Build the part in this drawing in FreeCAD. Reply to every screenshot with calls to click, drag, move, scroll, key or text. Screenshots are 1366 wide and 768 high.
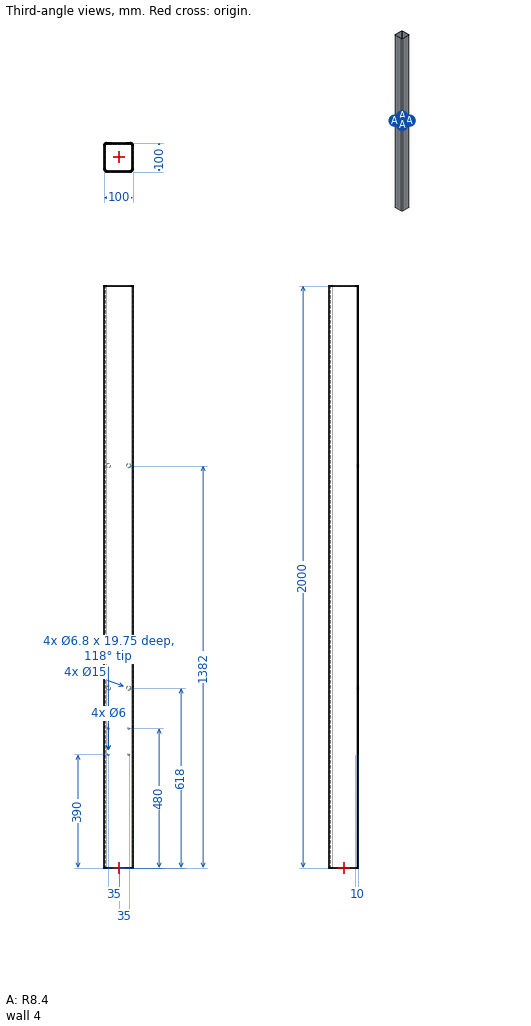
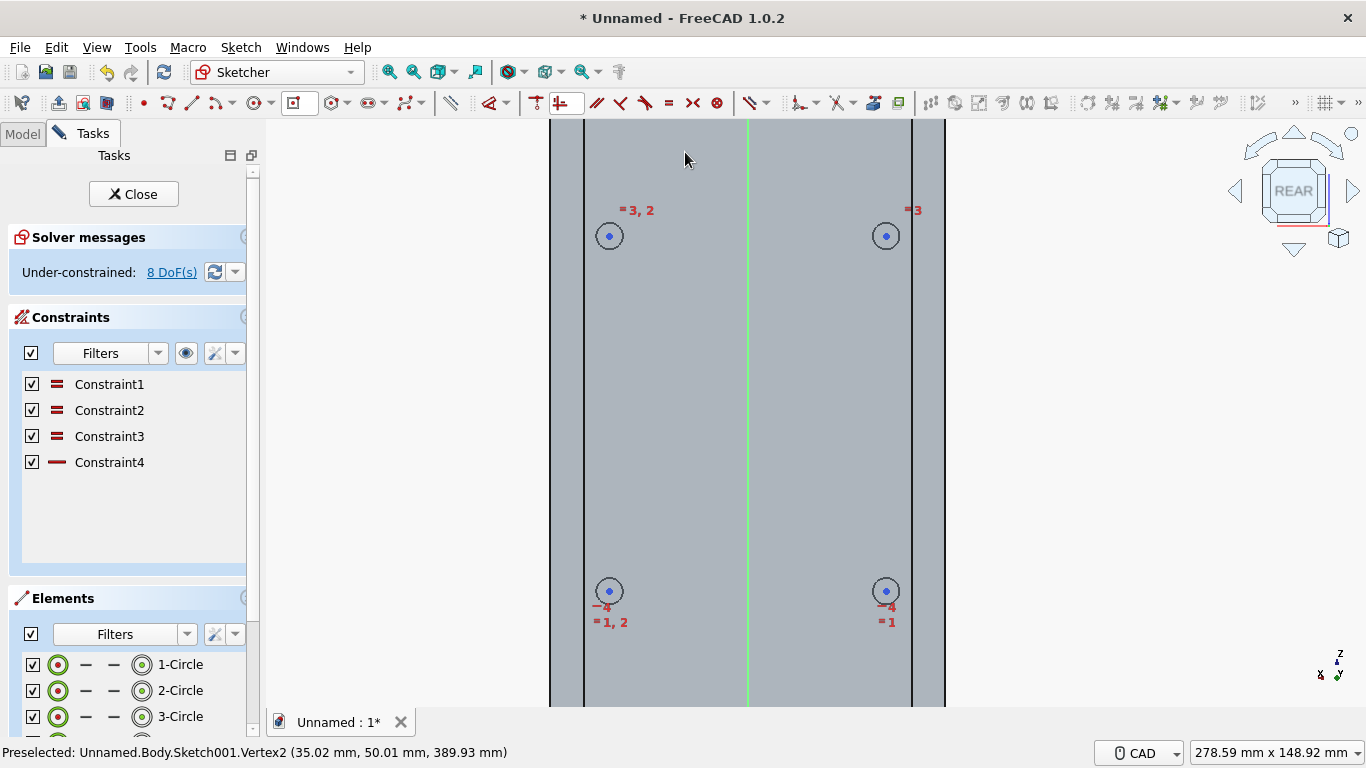
click(610, 591)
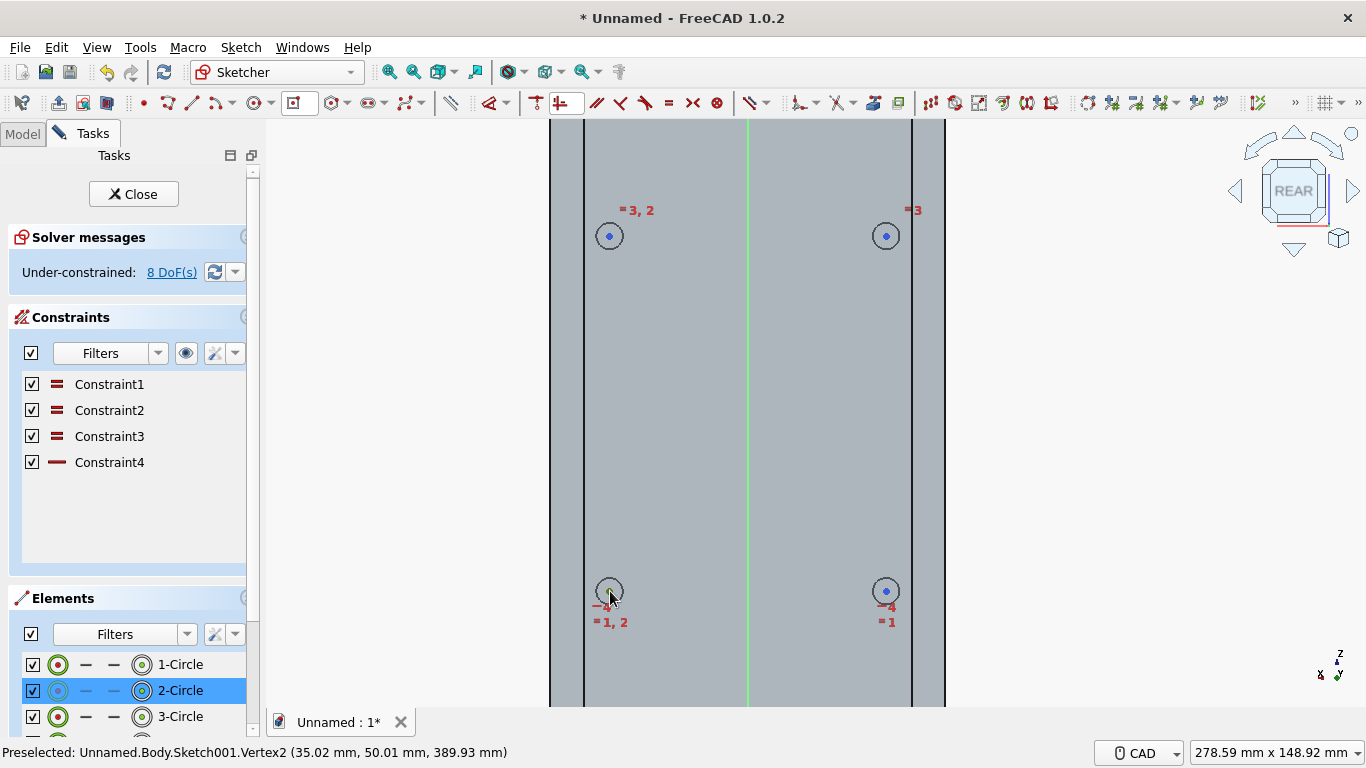
click(610, 236)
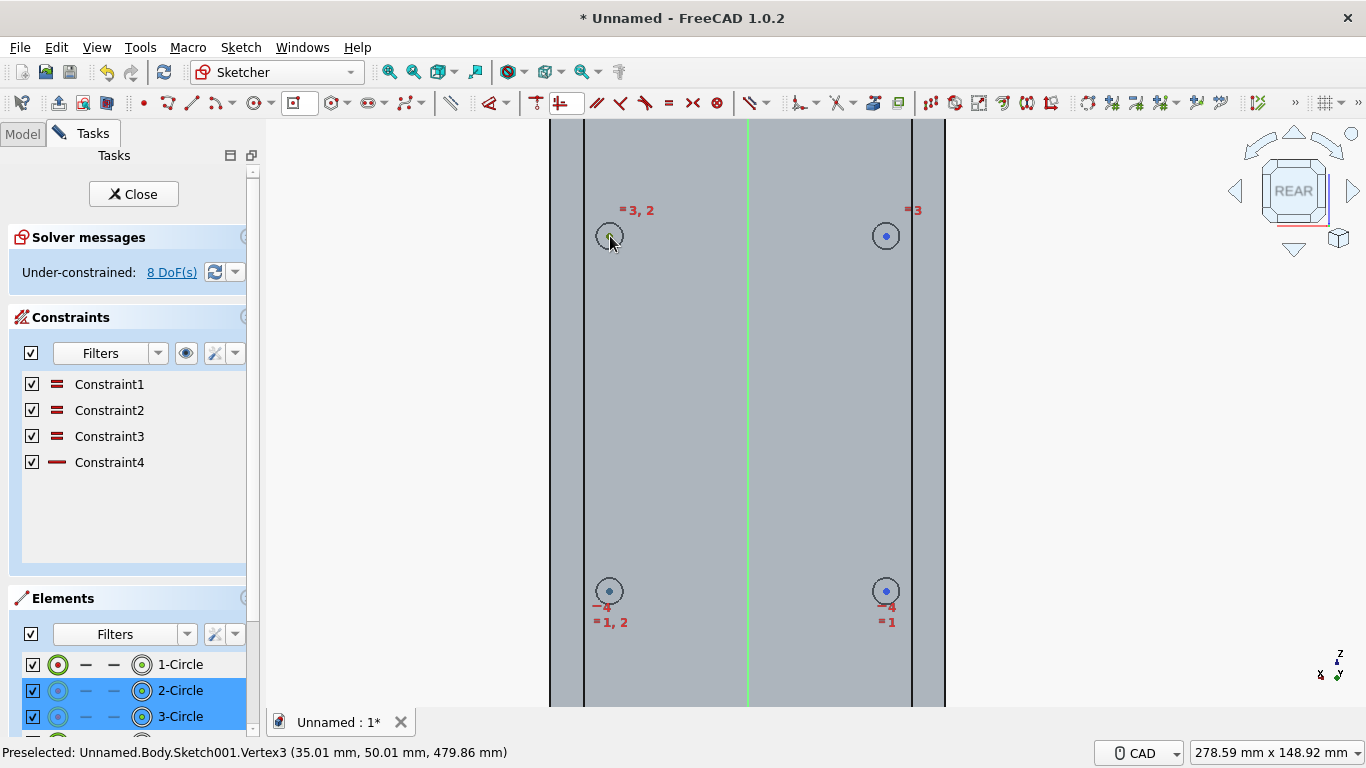
click(578, 104)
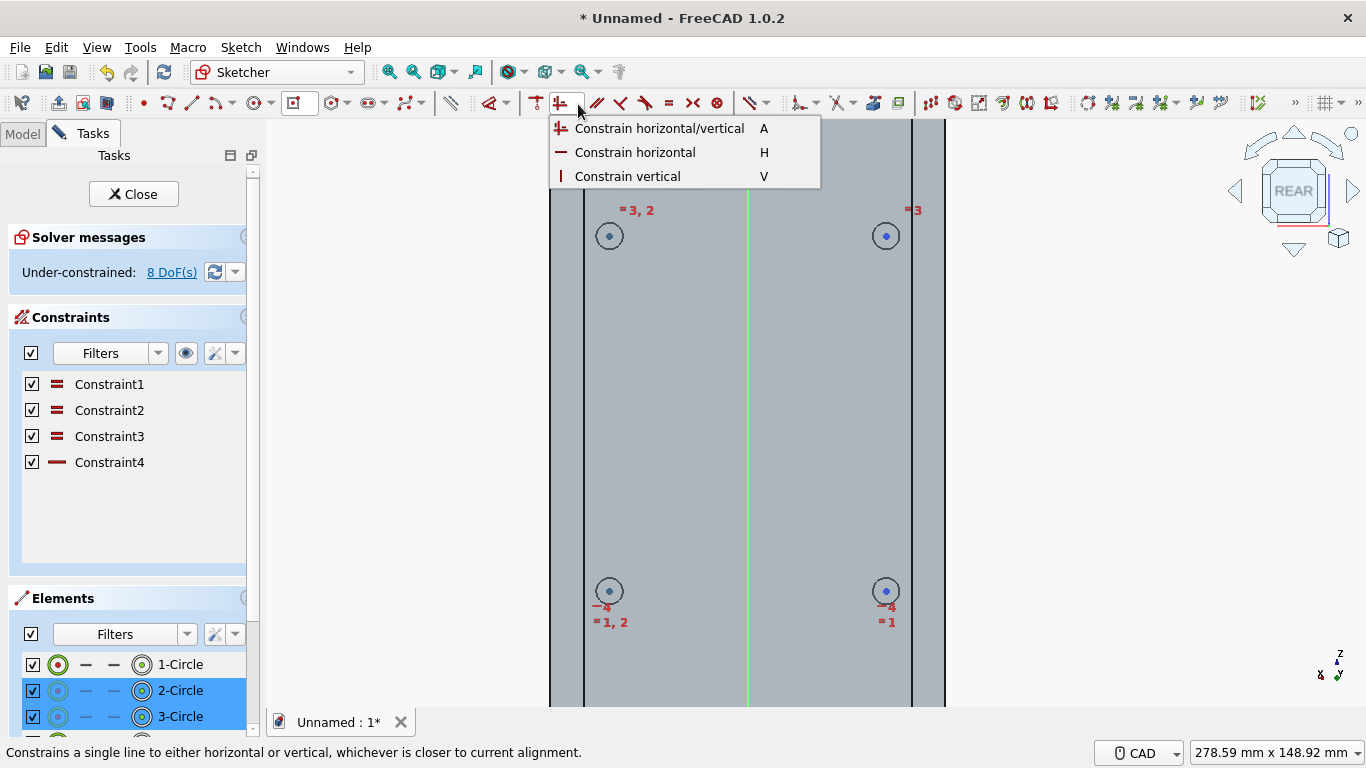
click(685, 176)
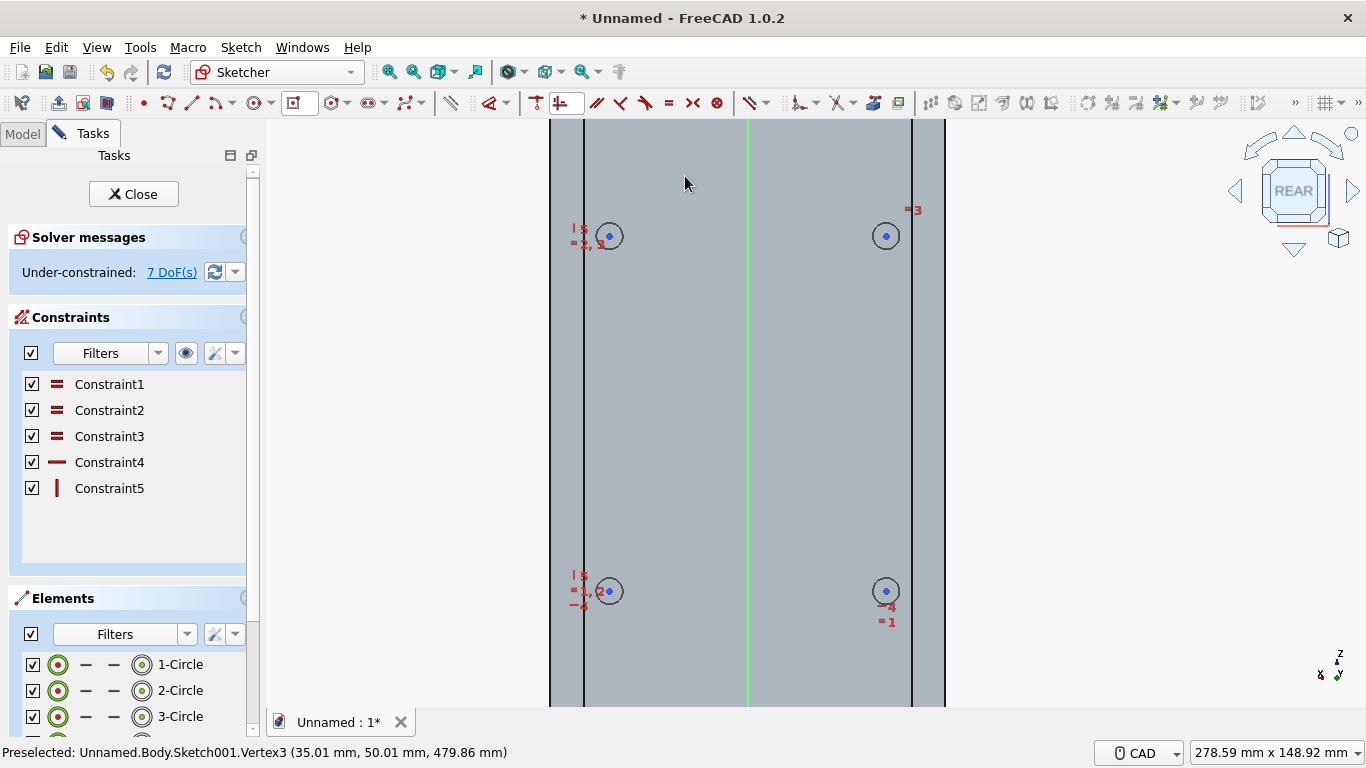
click(886, 591)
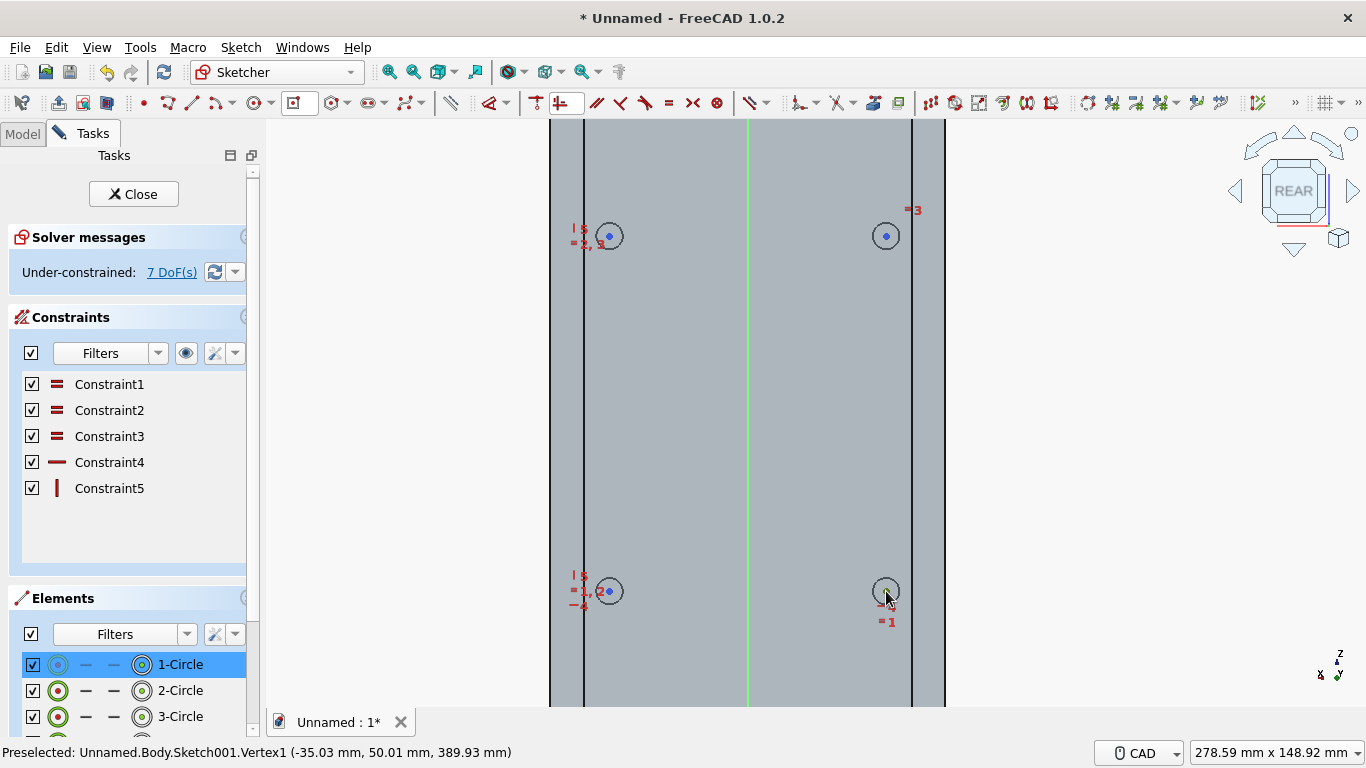
click(886, 236)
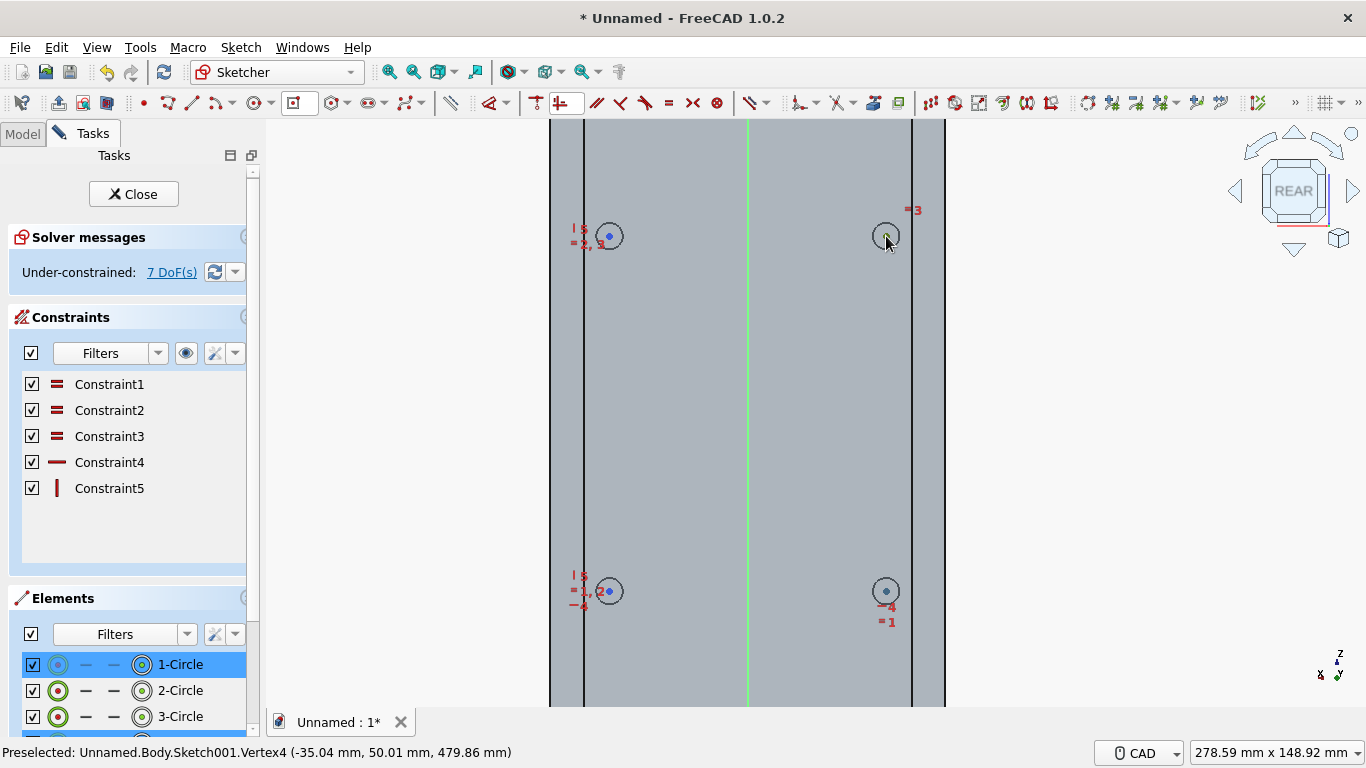
click(578, 104)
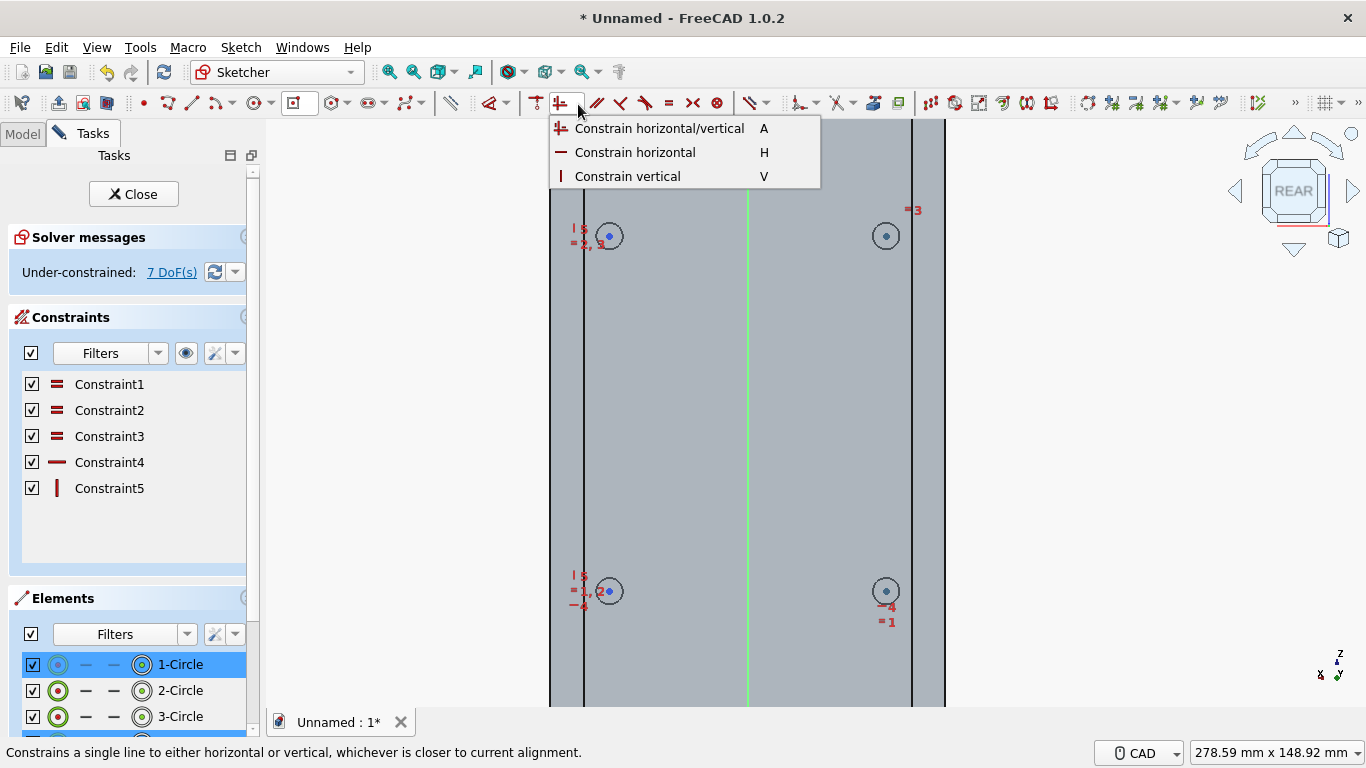
click(685, 176)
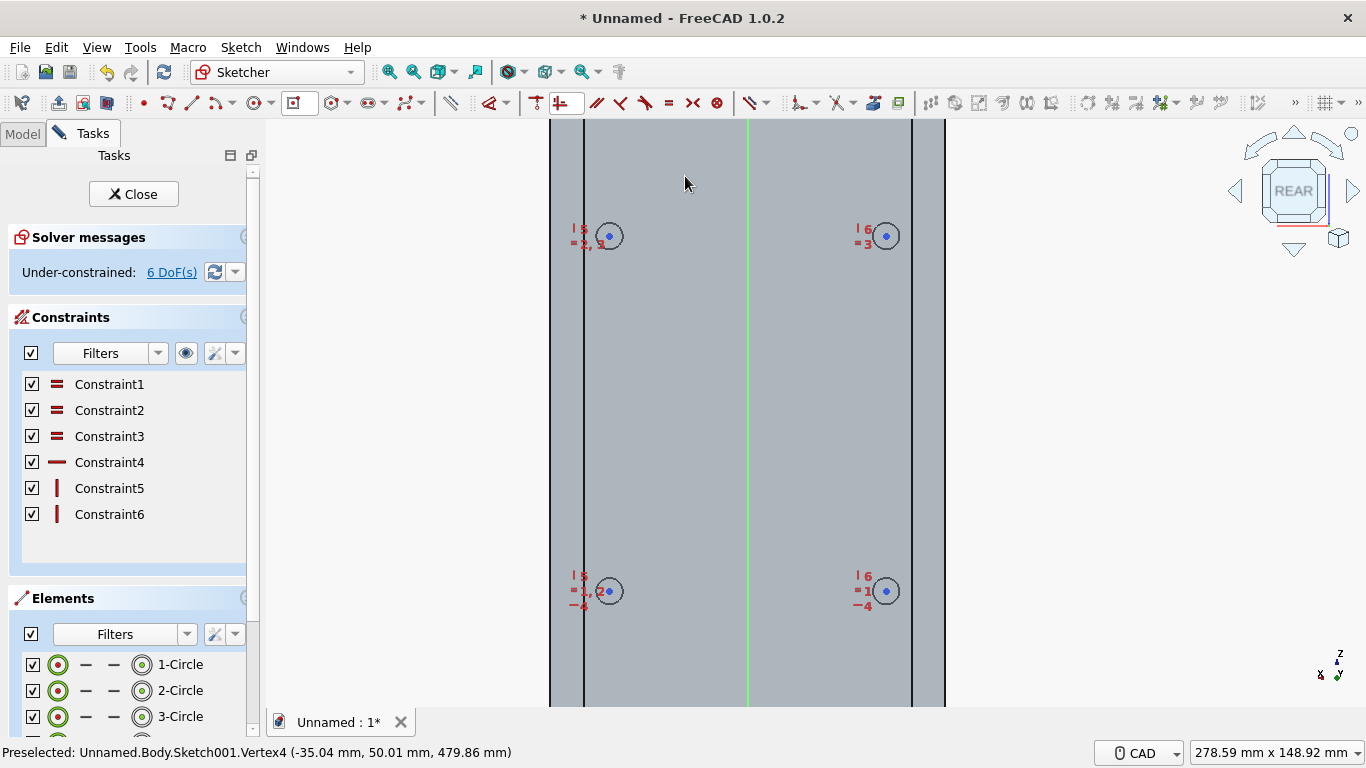
click(610, 236)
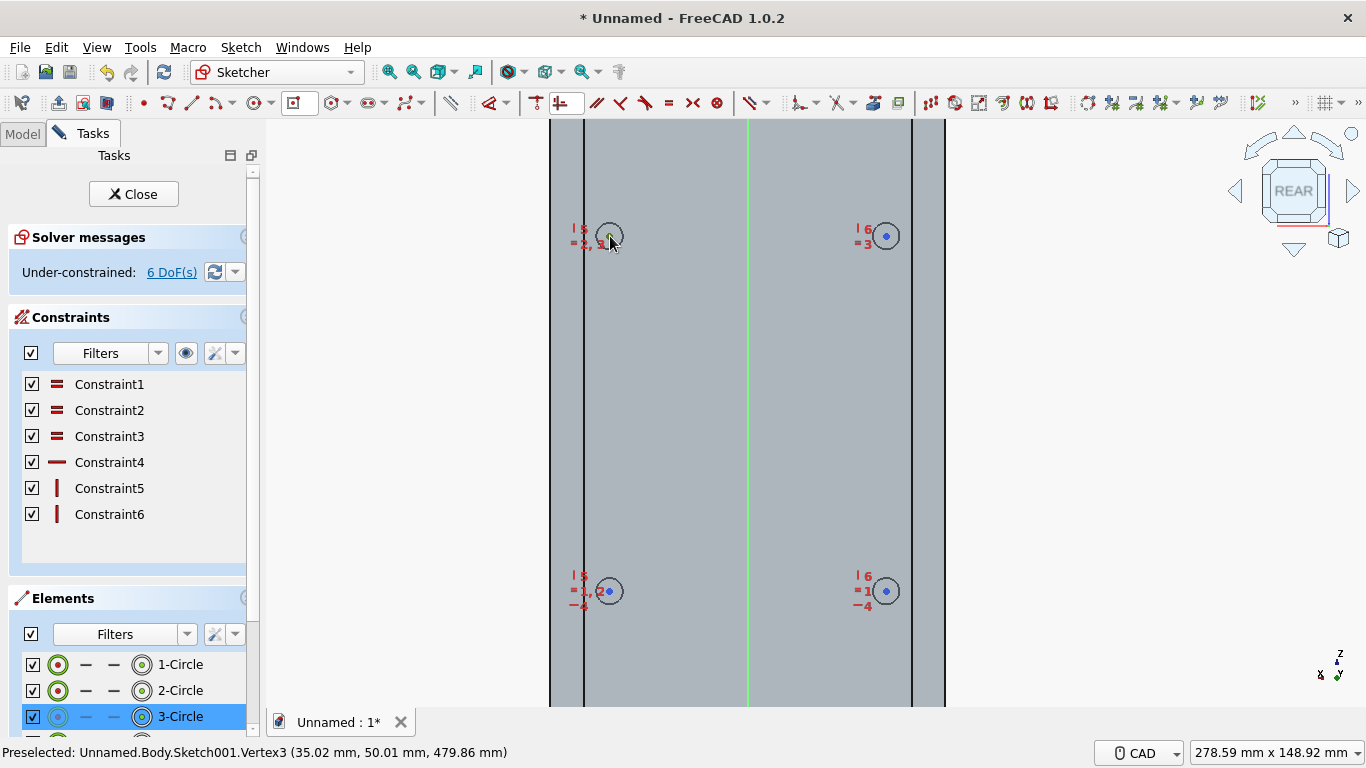
click(886, 236)